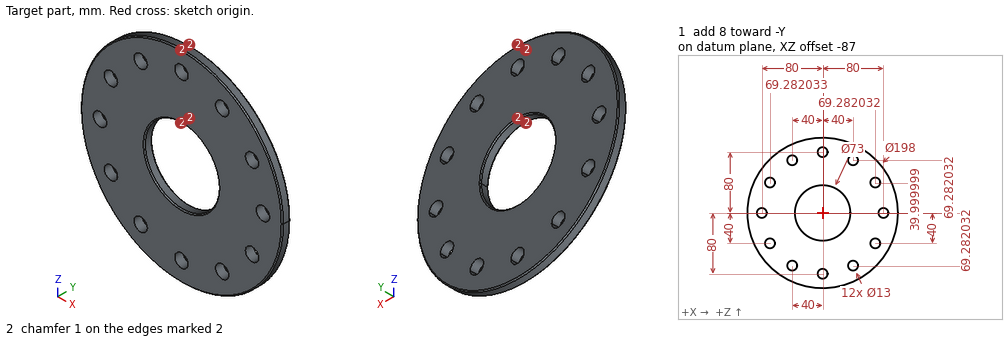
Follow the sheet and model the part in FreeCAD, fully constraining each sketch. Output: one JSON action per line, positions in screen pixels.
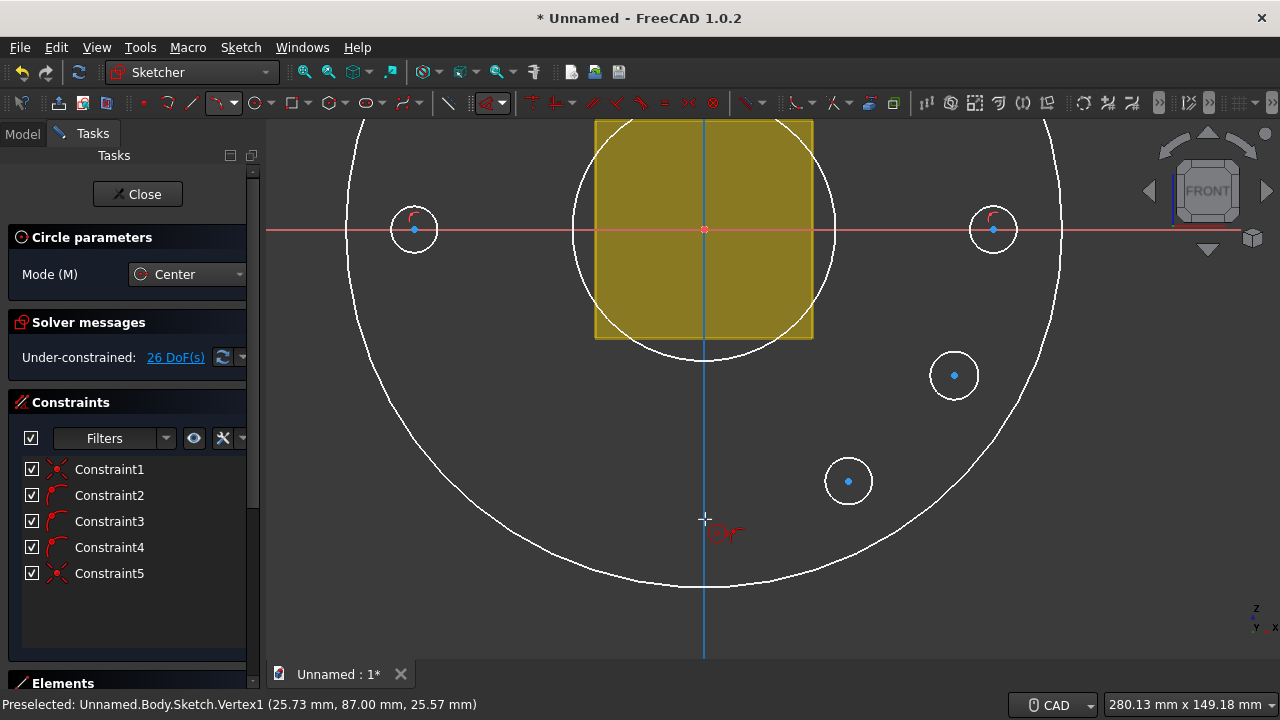
{"action": "left_click", "coordinate": [704, 519]}
{"action": "left_click", "coordinate": [721, 502]}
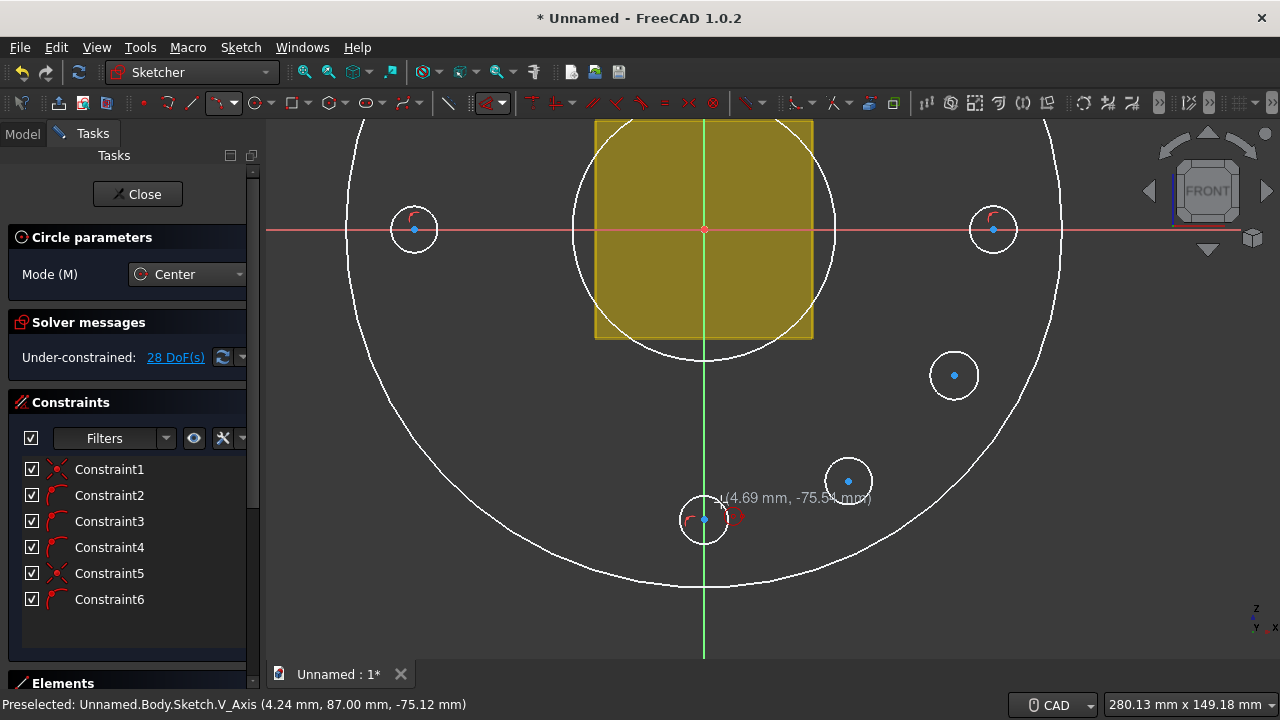
{"action": "left_click", "coordinate": [559, 480]}
{"action": "left_click", "coordinate": [576, 464]}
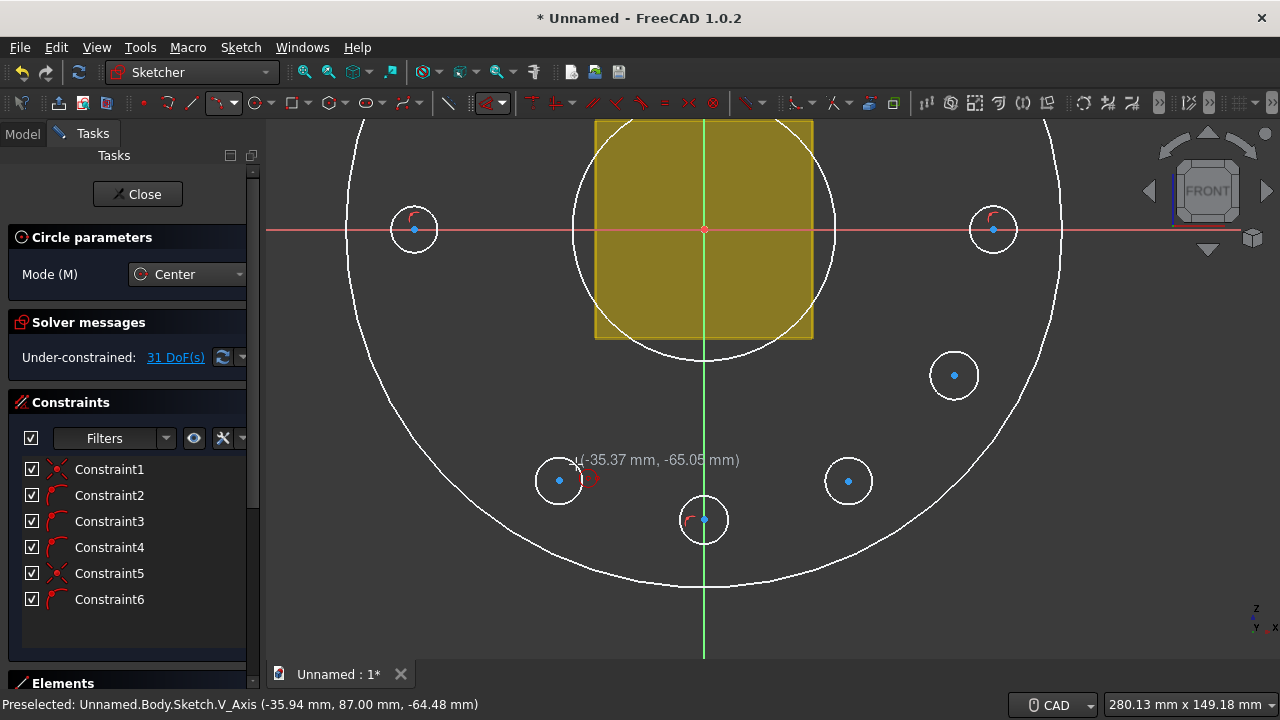
{"action": "left_click", "coordinate": [453, 374]}
{"action": "left_click", "coordinate": [470, 358]}
{"action": "key", "text": "Escape"}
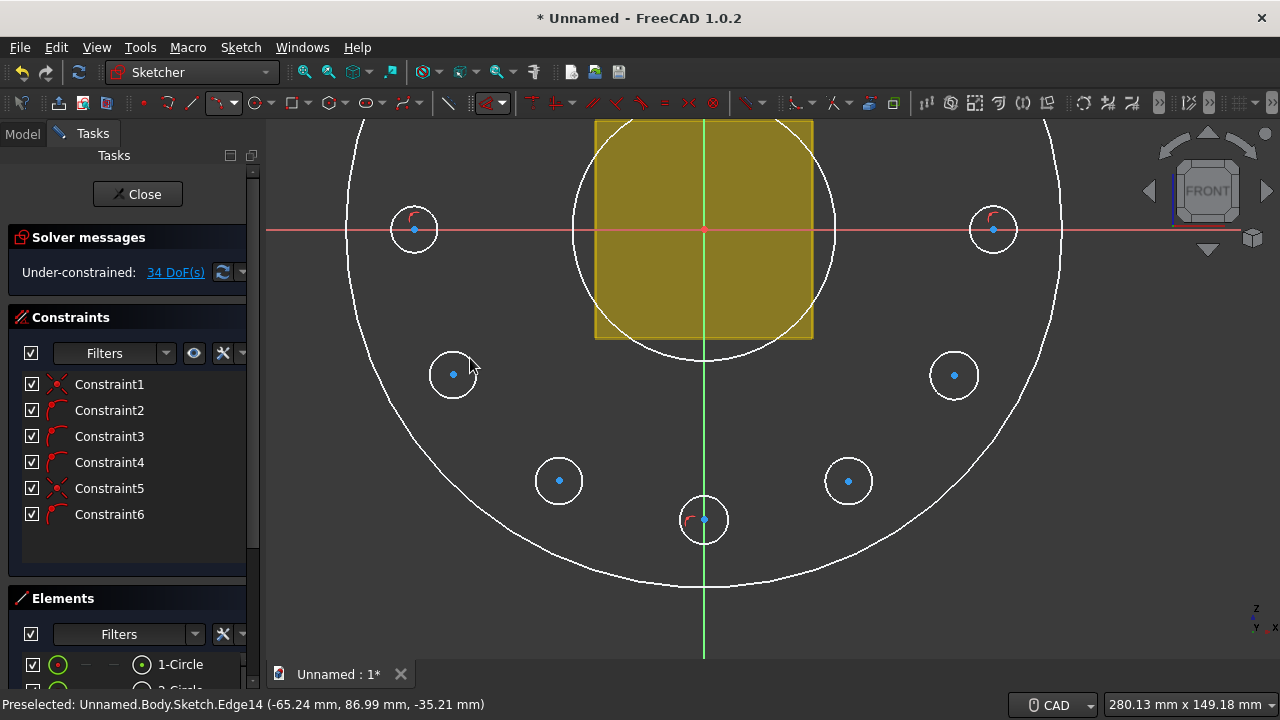
{"action": "scroll", "coordinate": [705, 519], "scroll_direction": "down", "scroll_amount": 4}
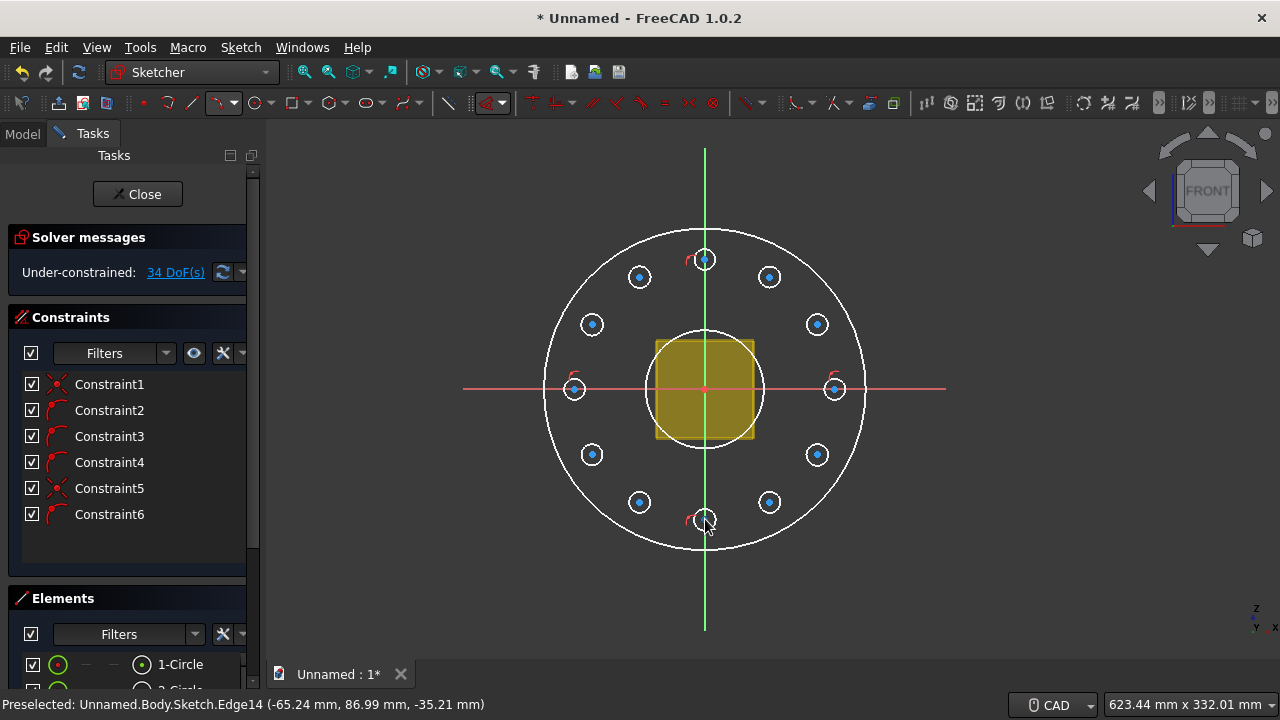
{"action": "scroll", "coordinate": [825, 317], "scroll_direction": "up", "scroll_amount": 2}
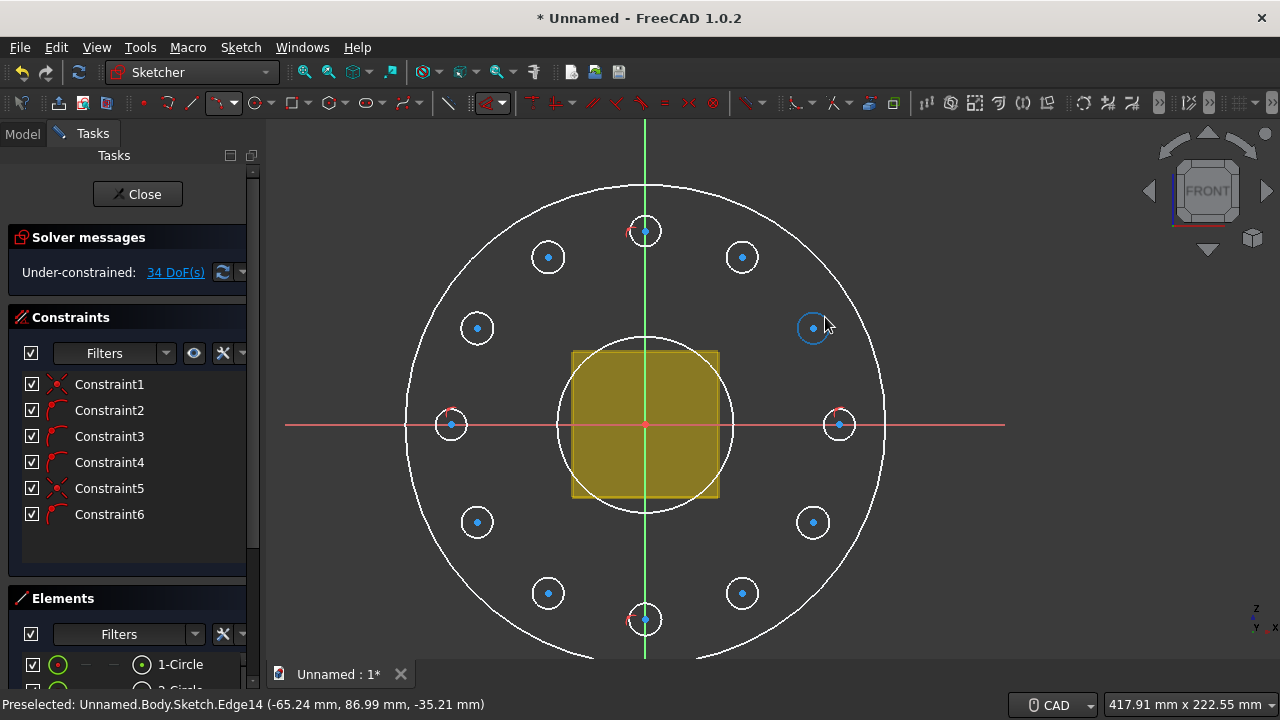
{"action": "left_click", "coordinate": [824, 317]}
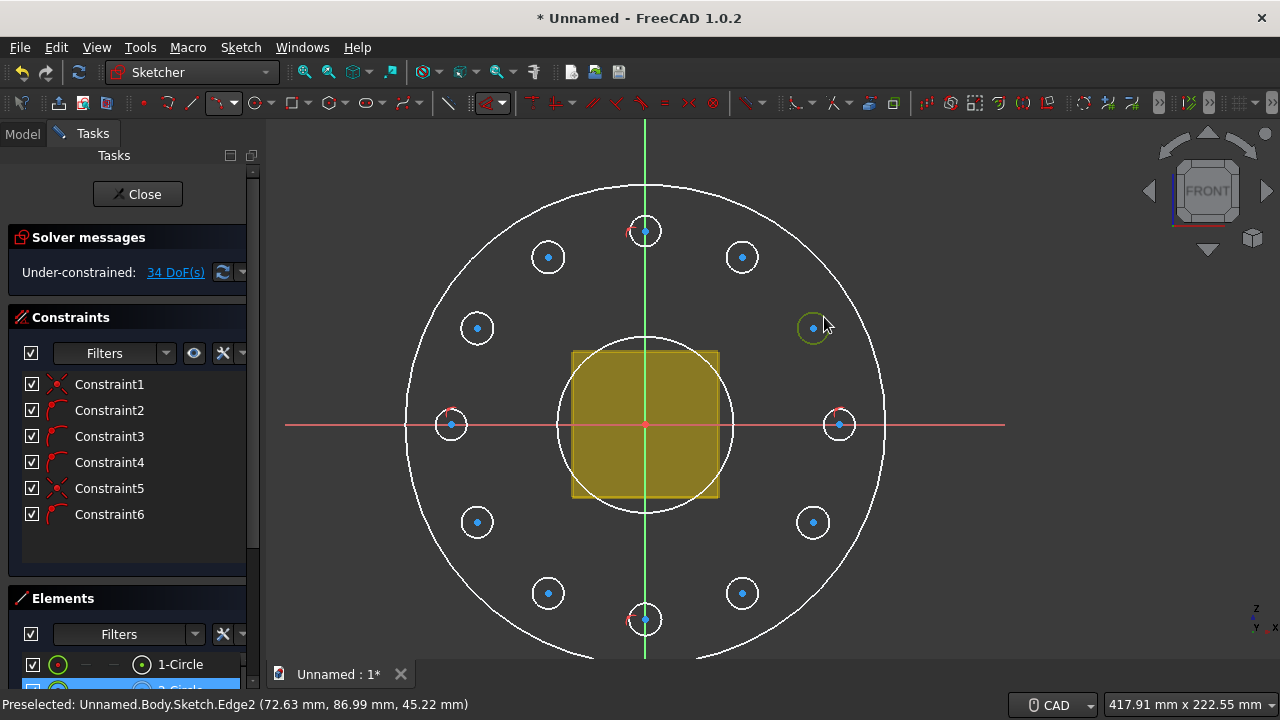
{"action": "left_click", "coordinate": [753, 246]}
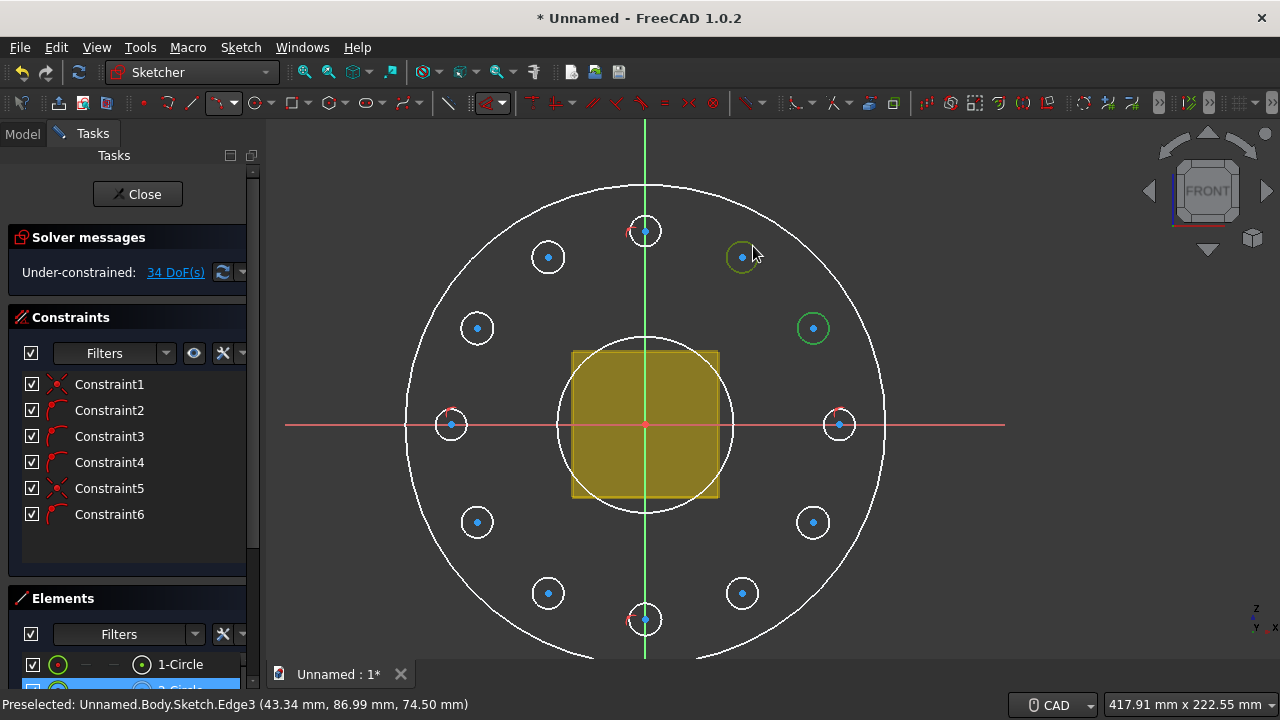
{"action": "scroll", "coordinate": [656, 220], "scroll_direction": "up", "scroll_amount": 2}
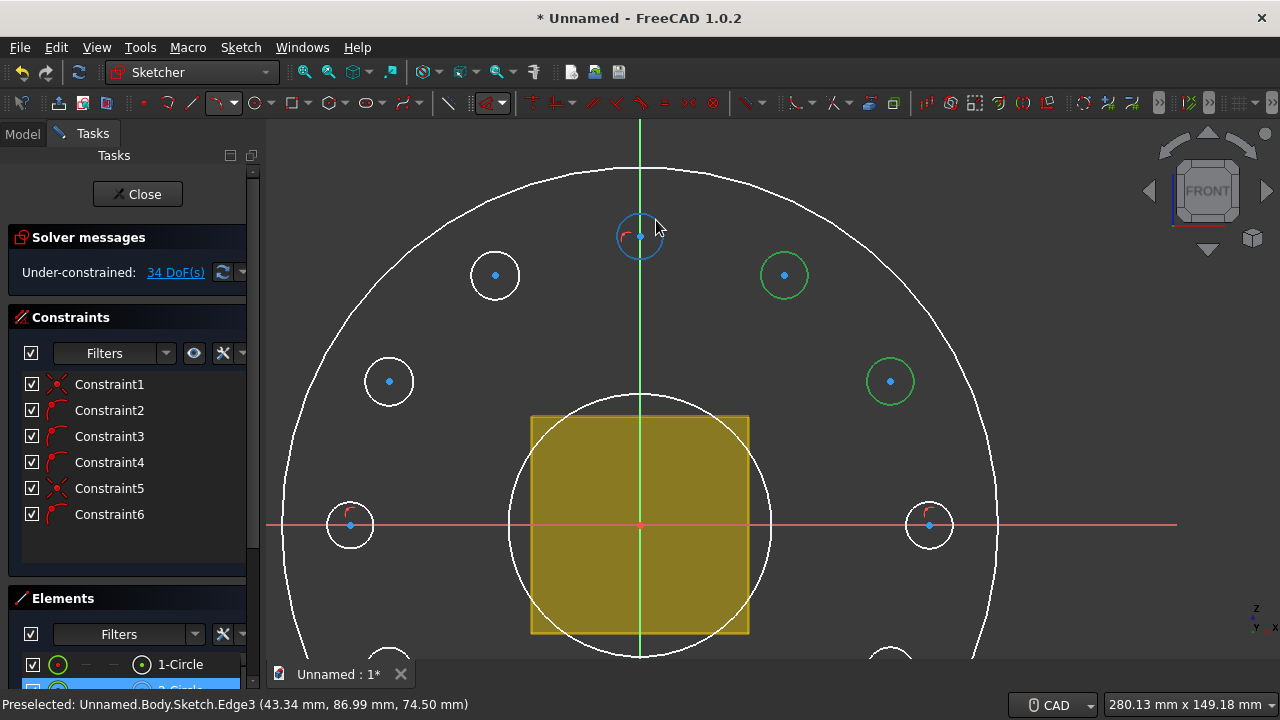
{"action": "left_click", "coordinate": [656, 220]}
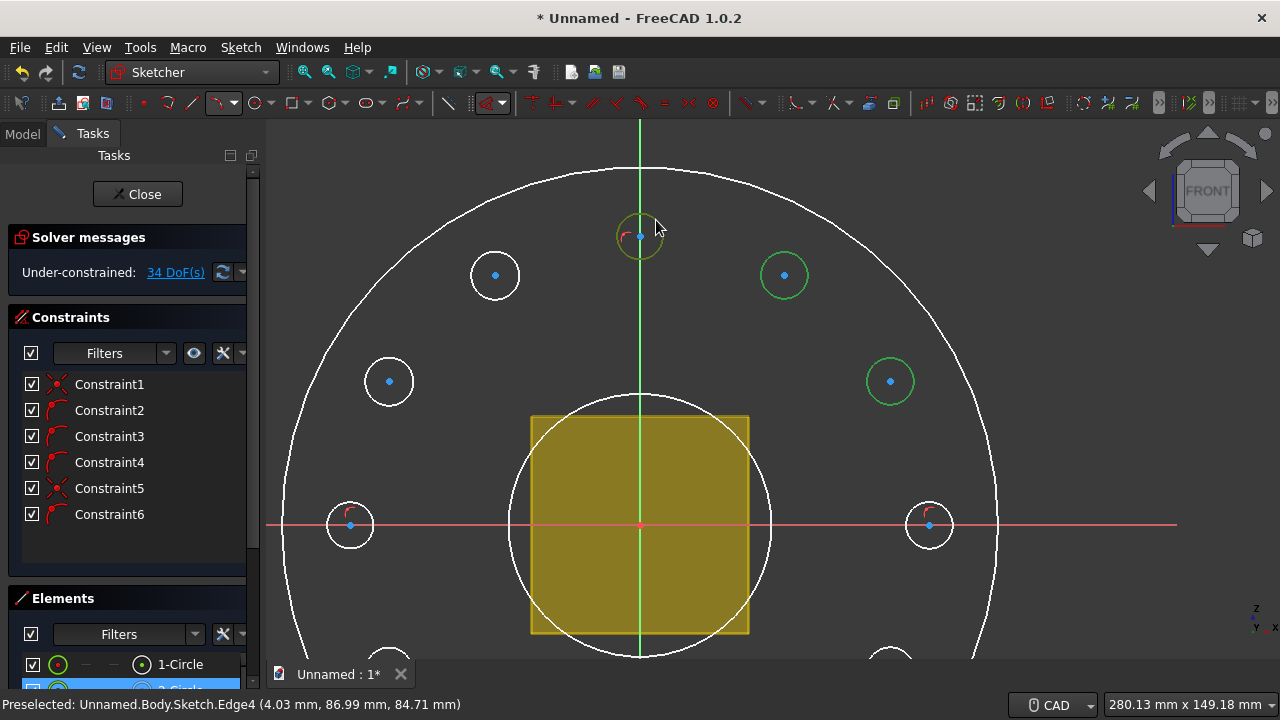
{"action": "left_click", "coordinate": [946, 509]}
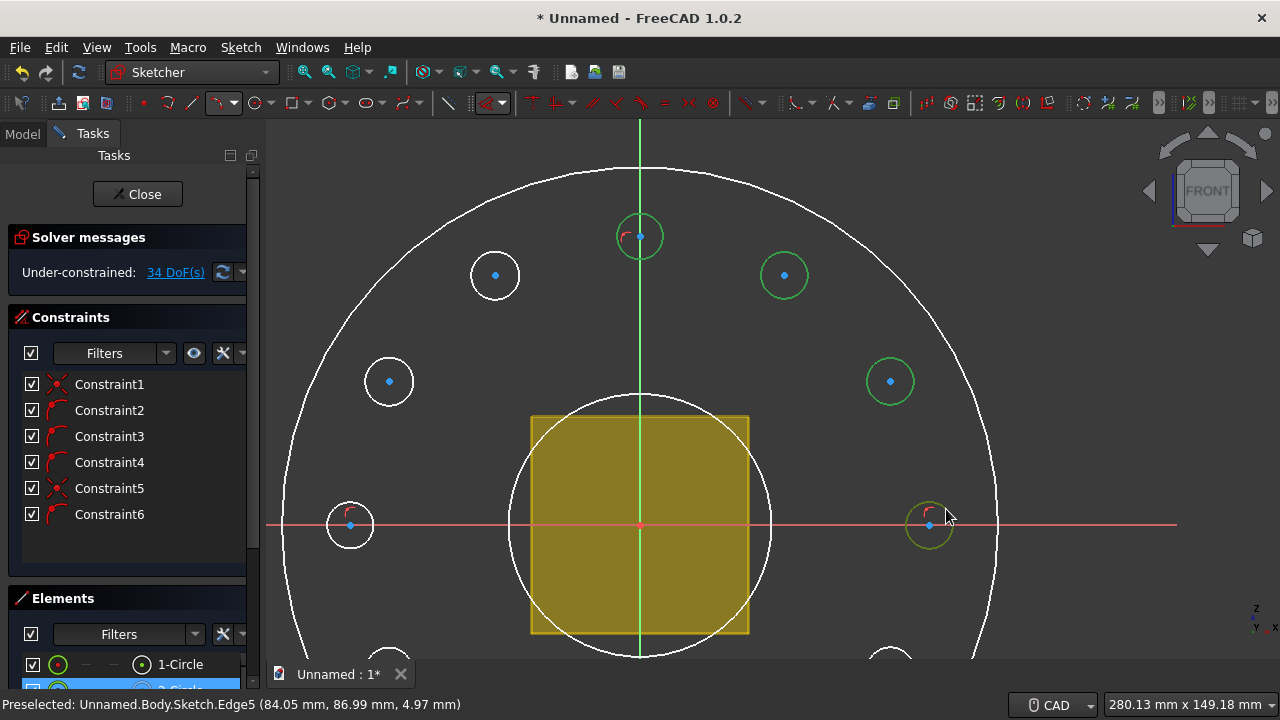
{"action": "scroll", "coordinate": [757, 278], "scroll_direction": "down", "scroll_amount": 4}